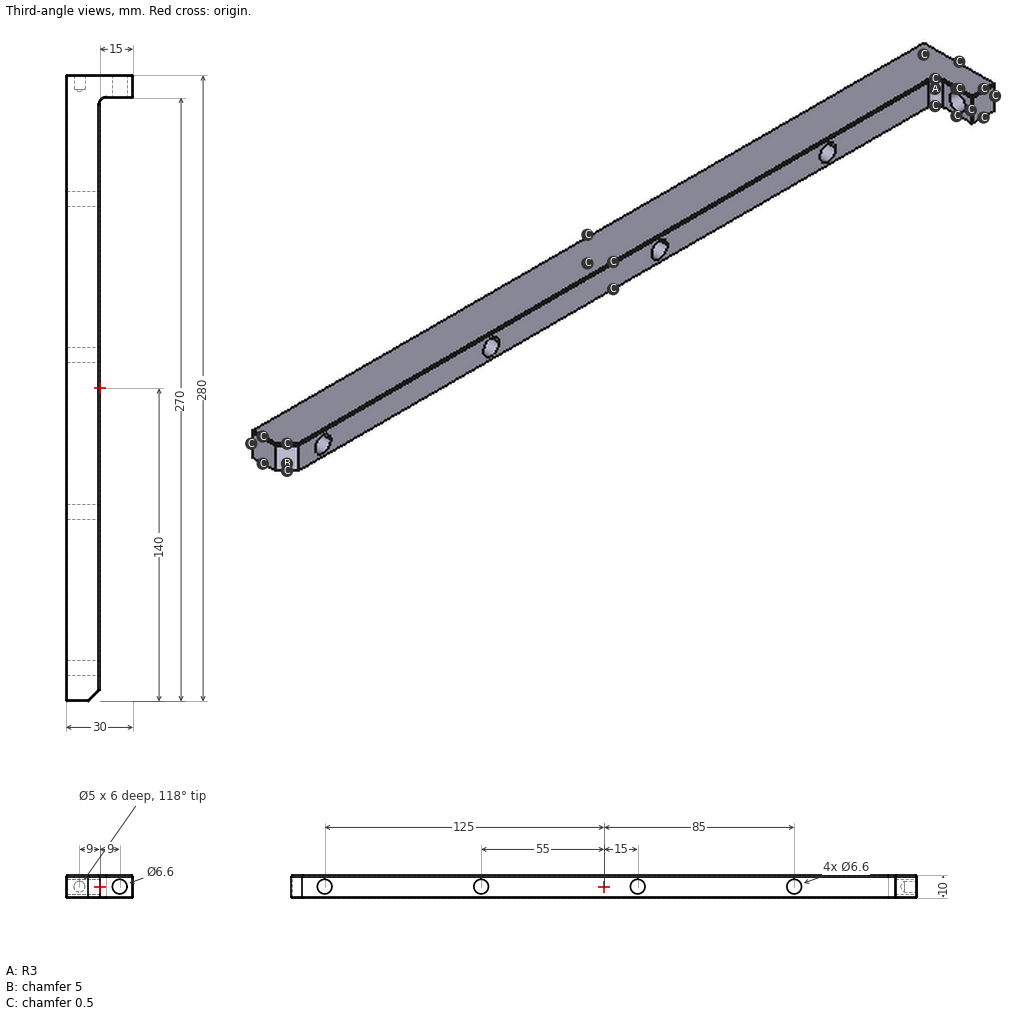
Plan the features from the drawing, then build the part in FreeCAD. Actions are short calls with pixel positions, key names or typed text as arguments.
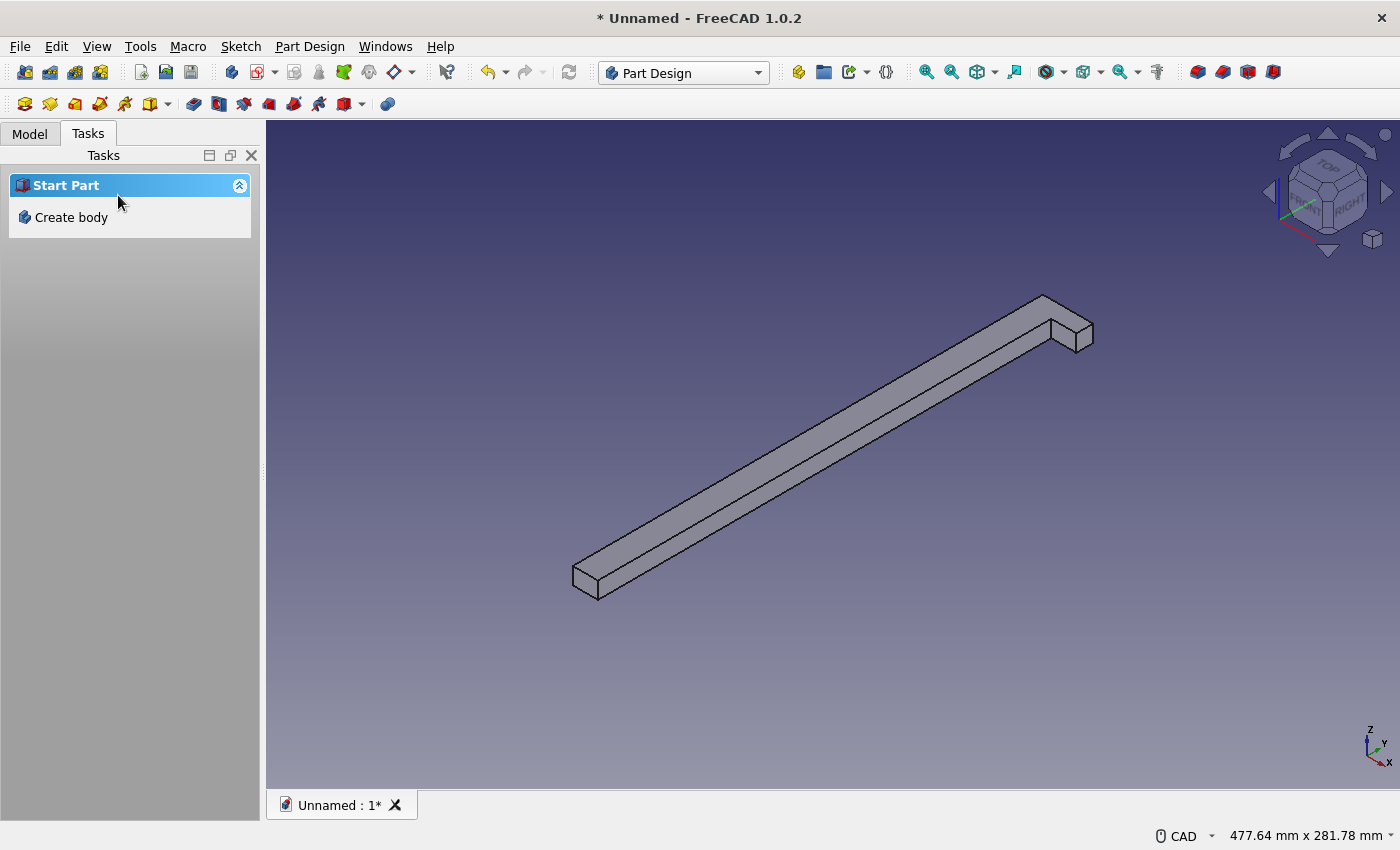
key(2)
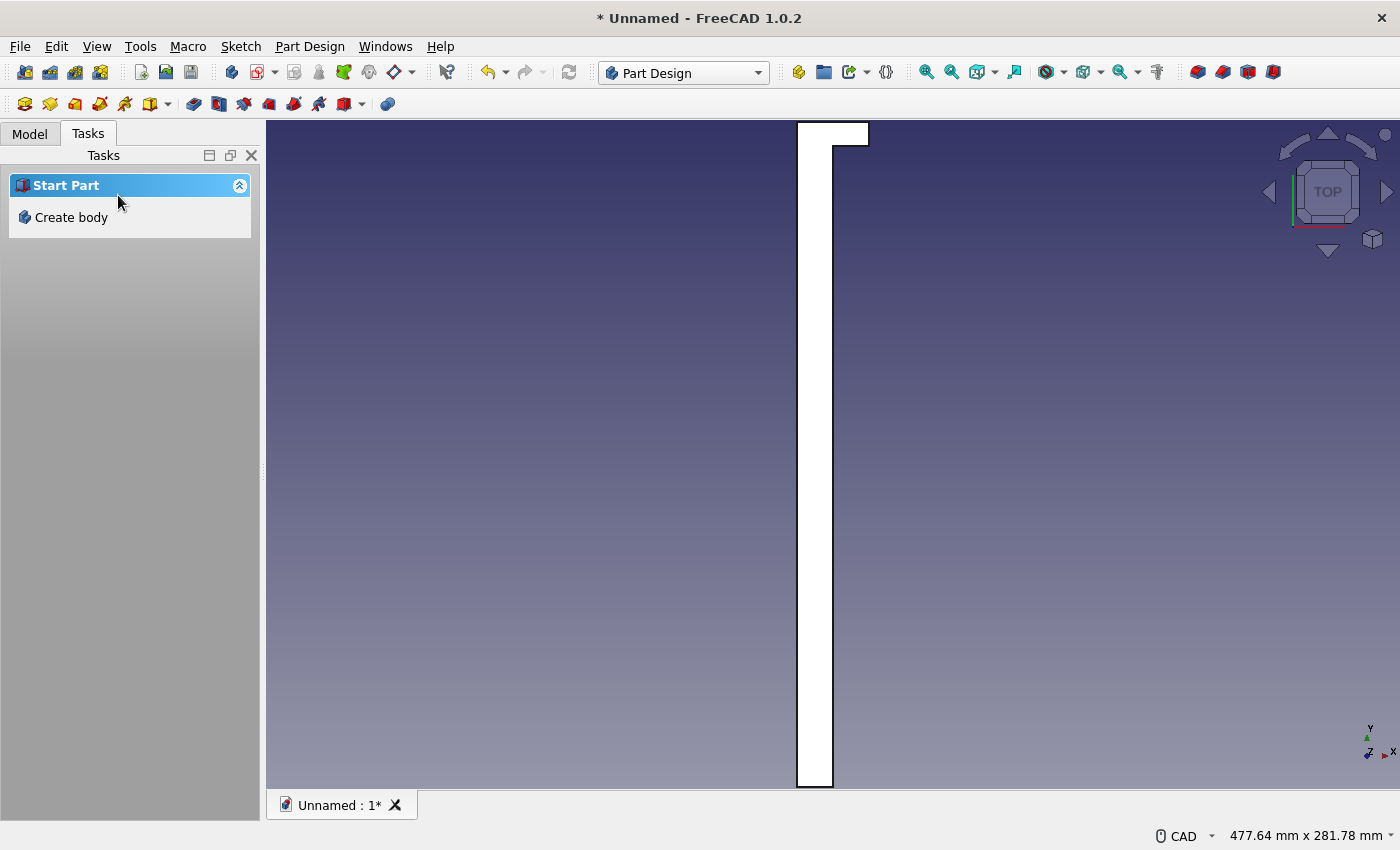
key(1)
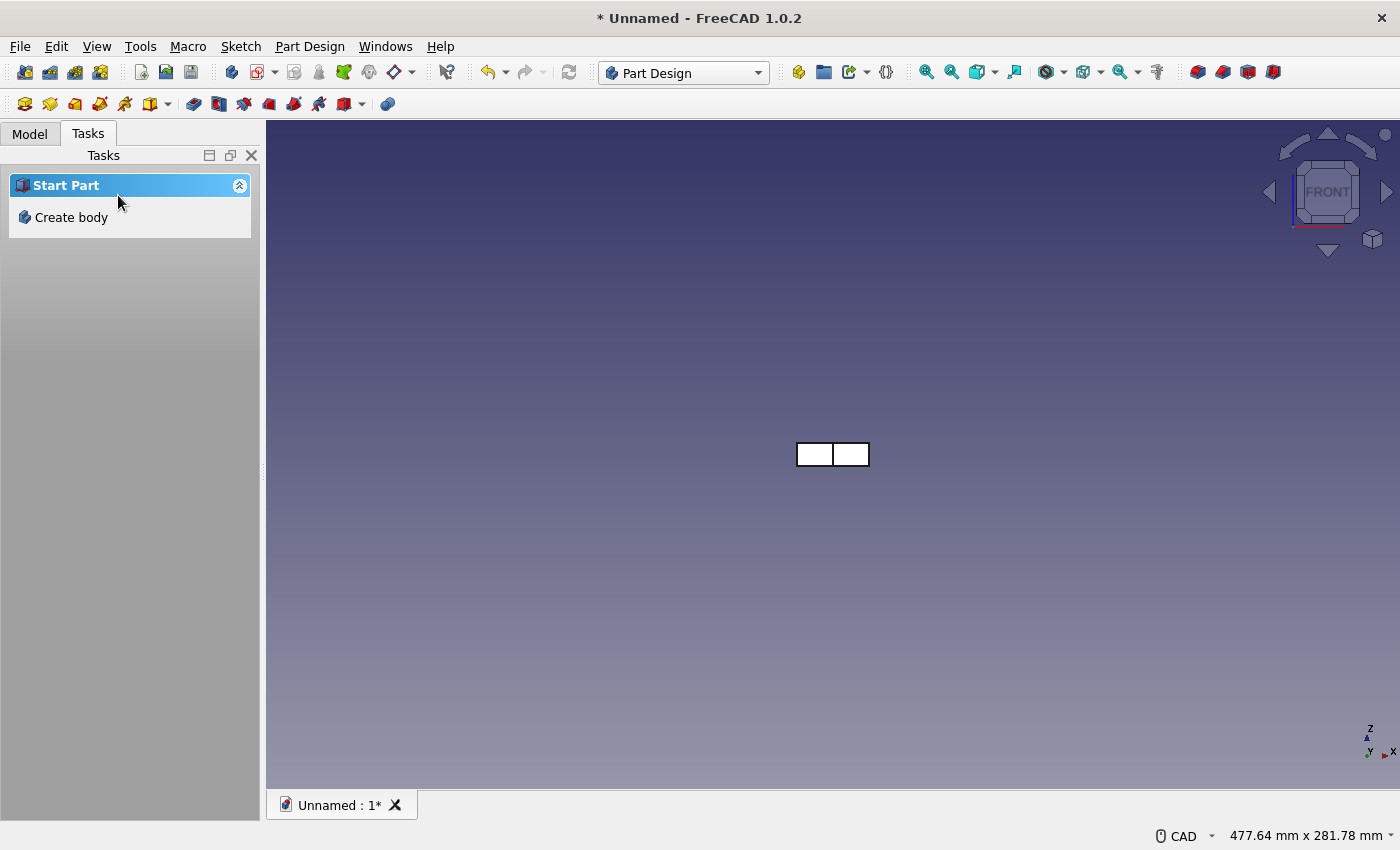
key(v)
key(f)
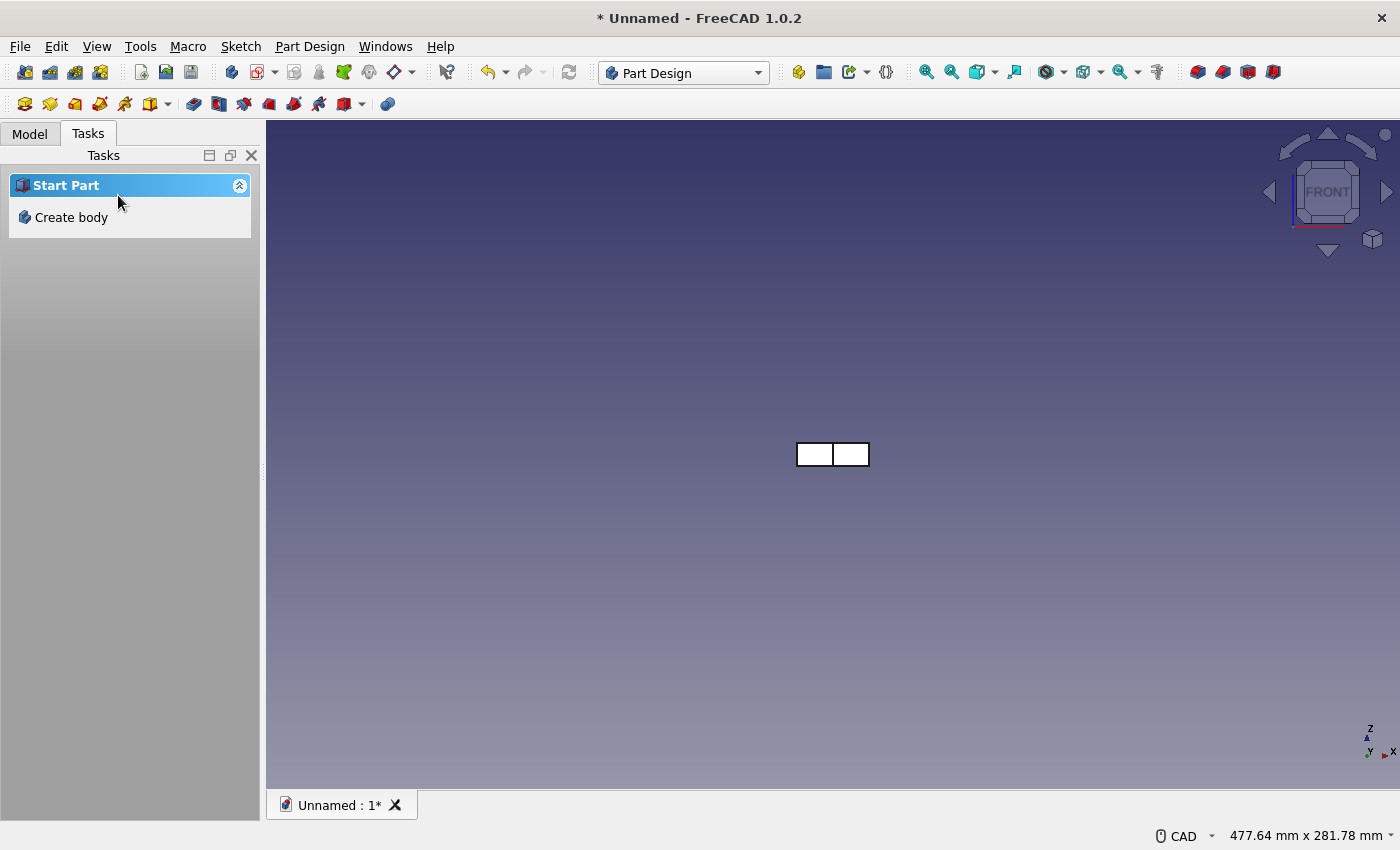
key(3)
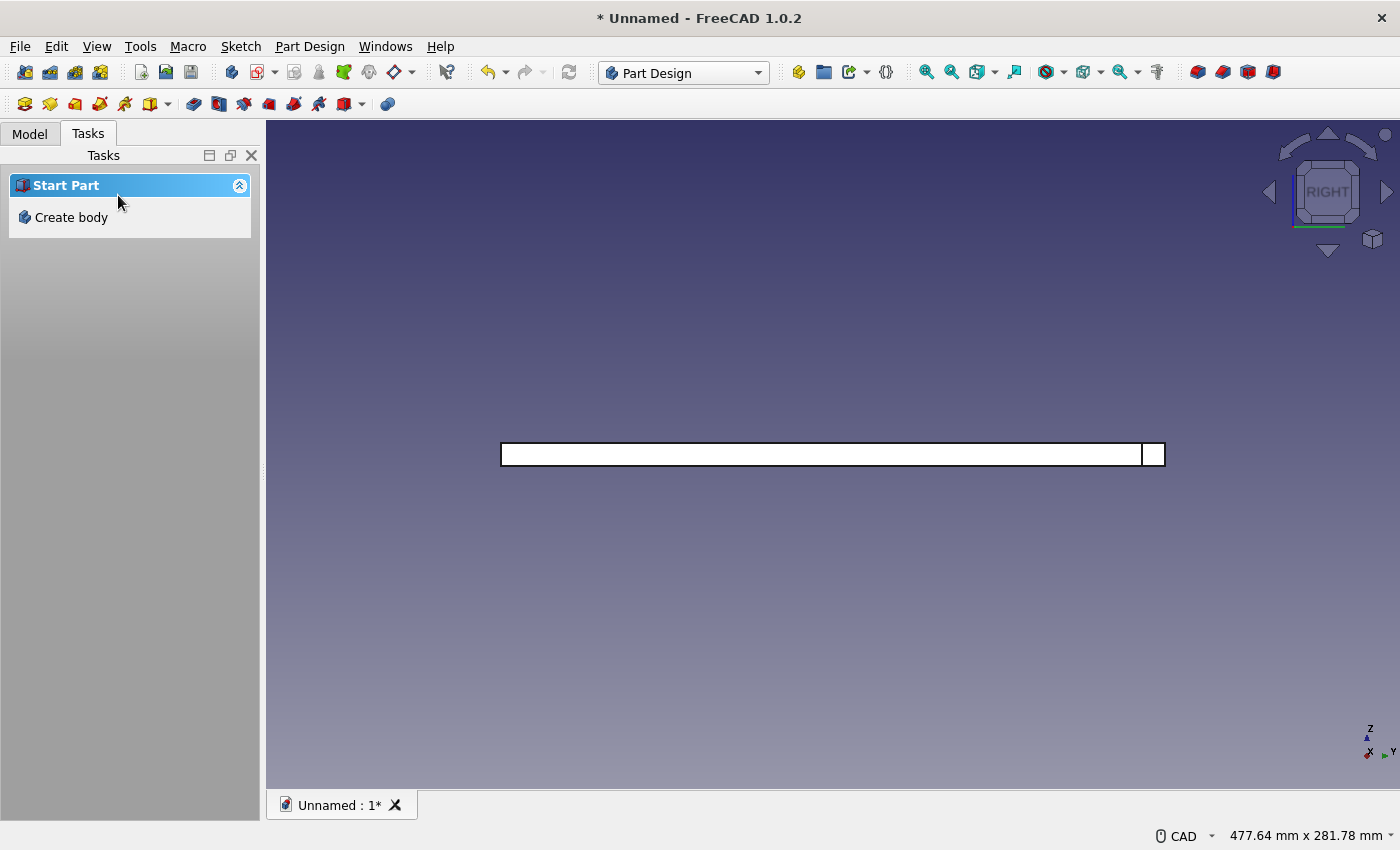
key(5)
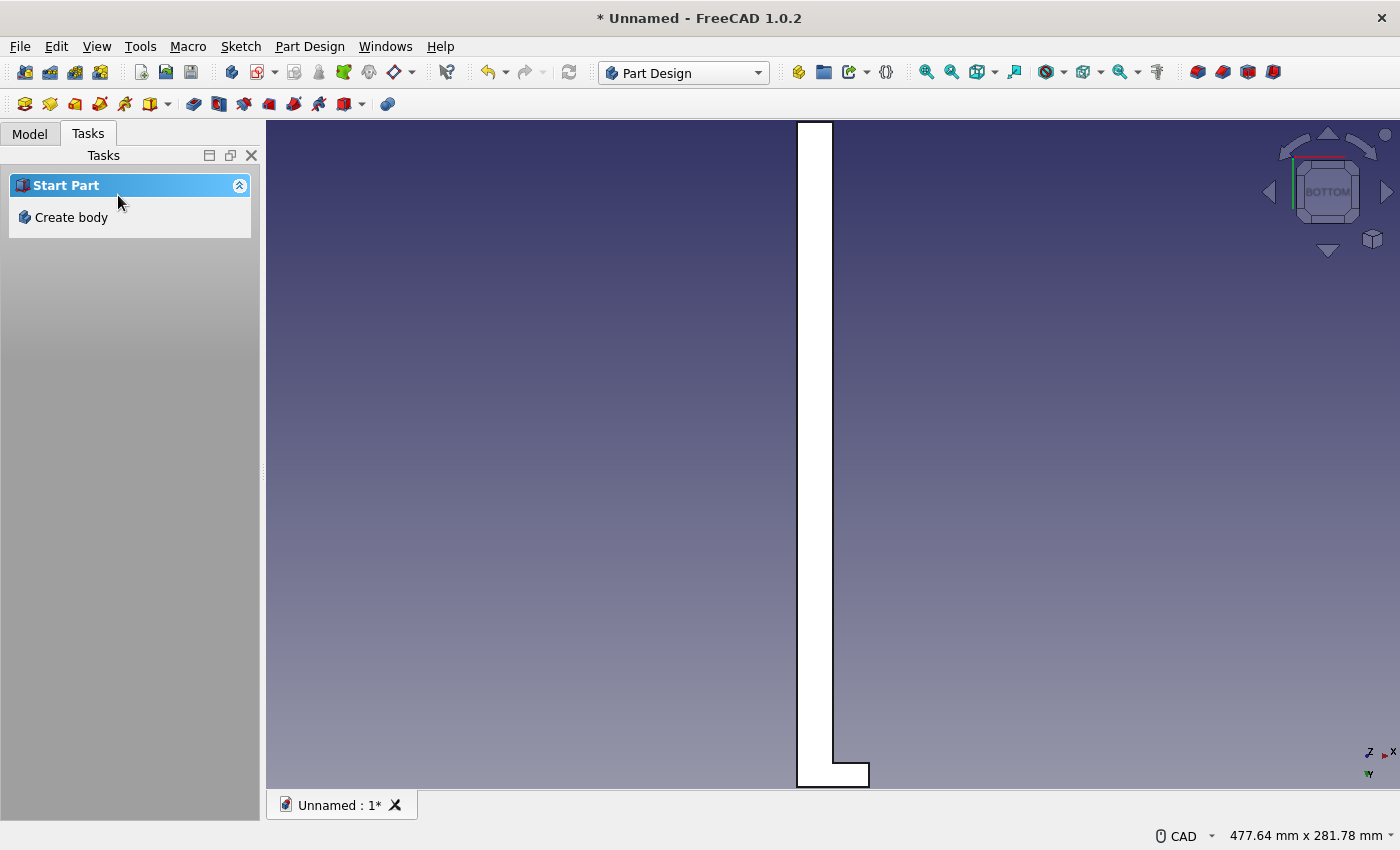
key(4)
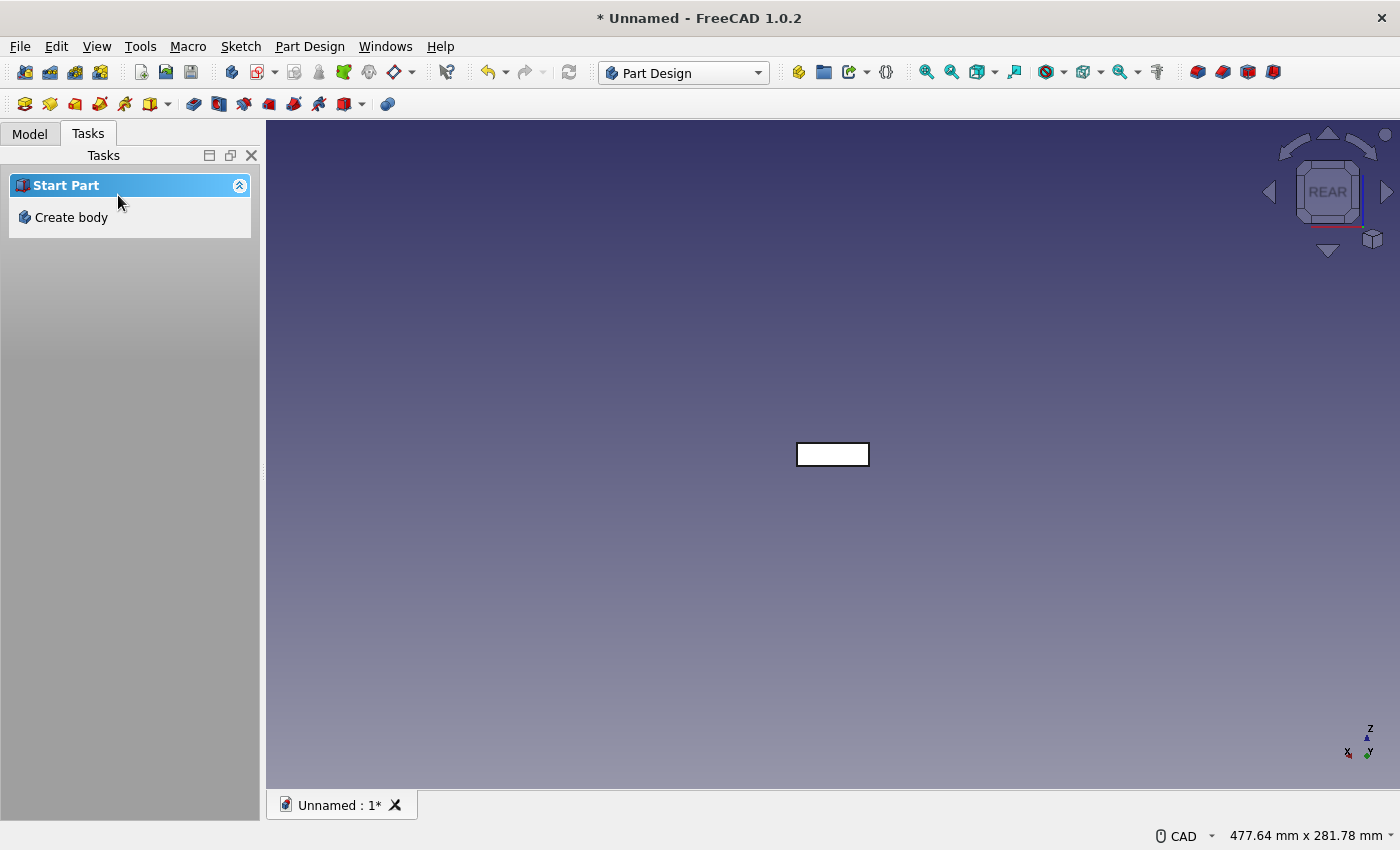
click(927, 72)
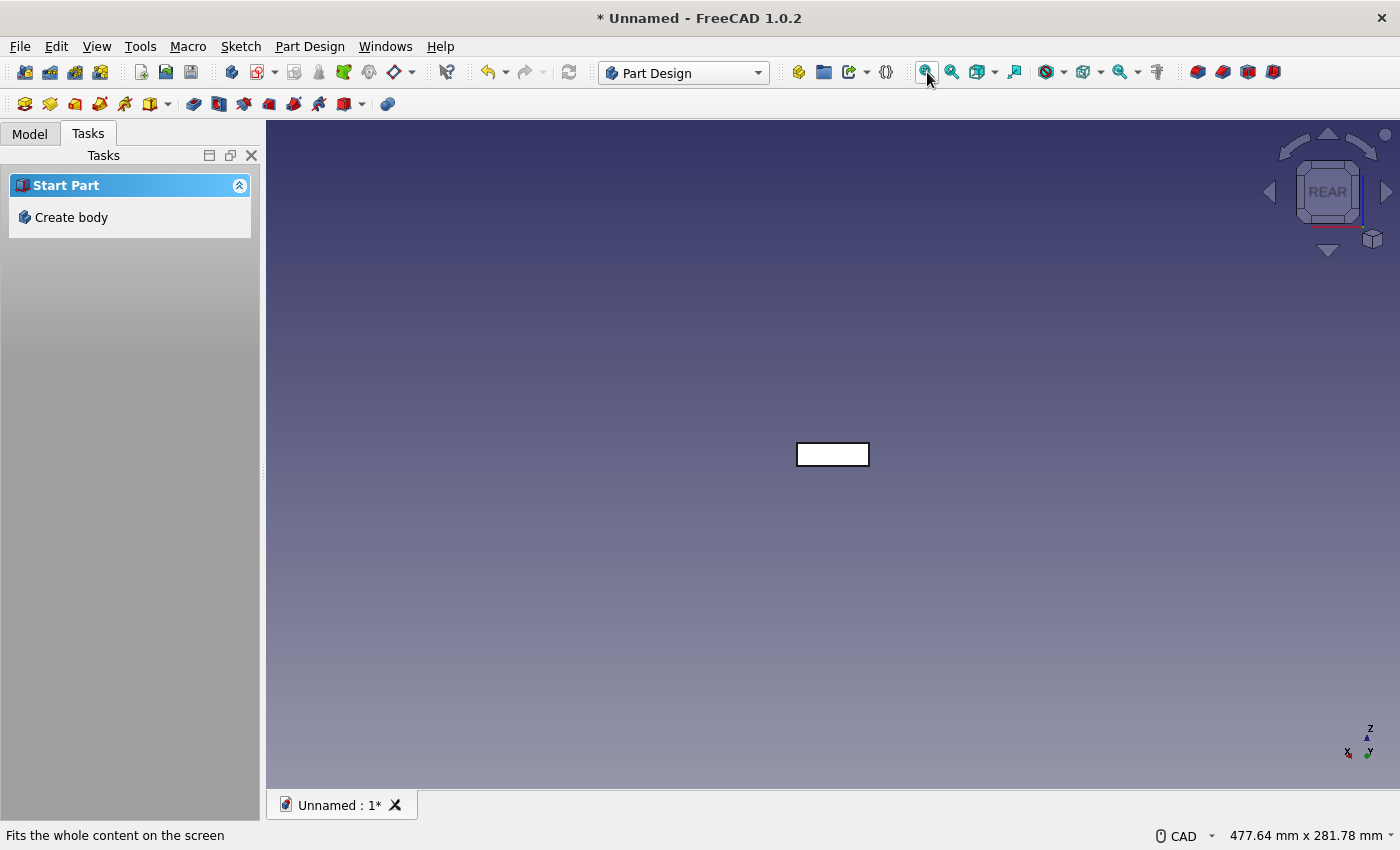
key(6)